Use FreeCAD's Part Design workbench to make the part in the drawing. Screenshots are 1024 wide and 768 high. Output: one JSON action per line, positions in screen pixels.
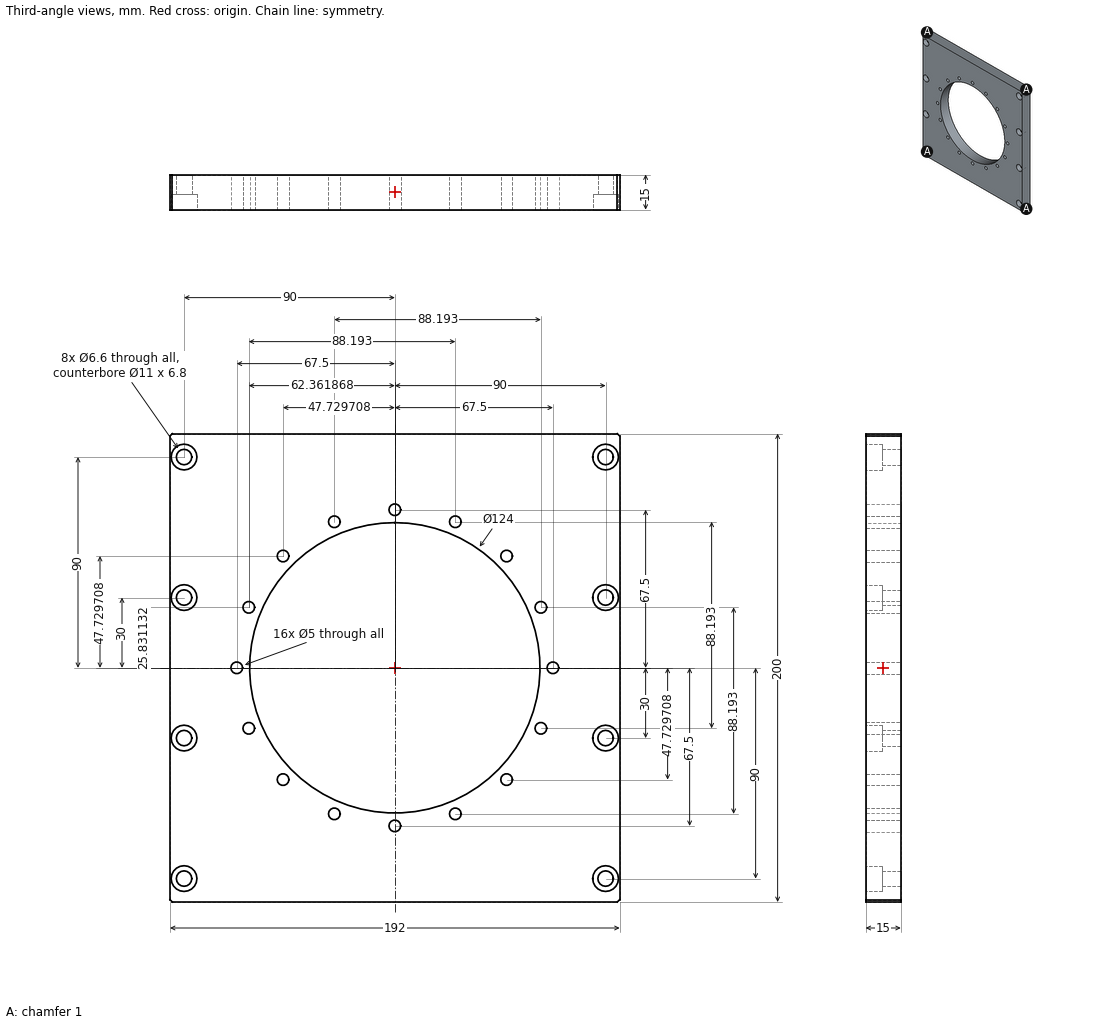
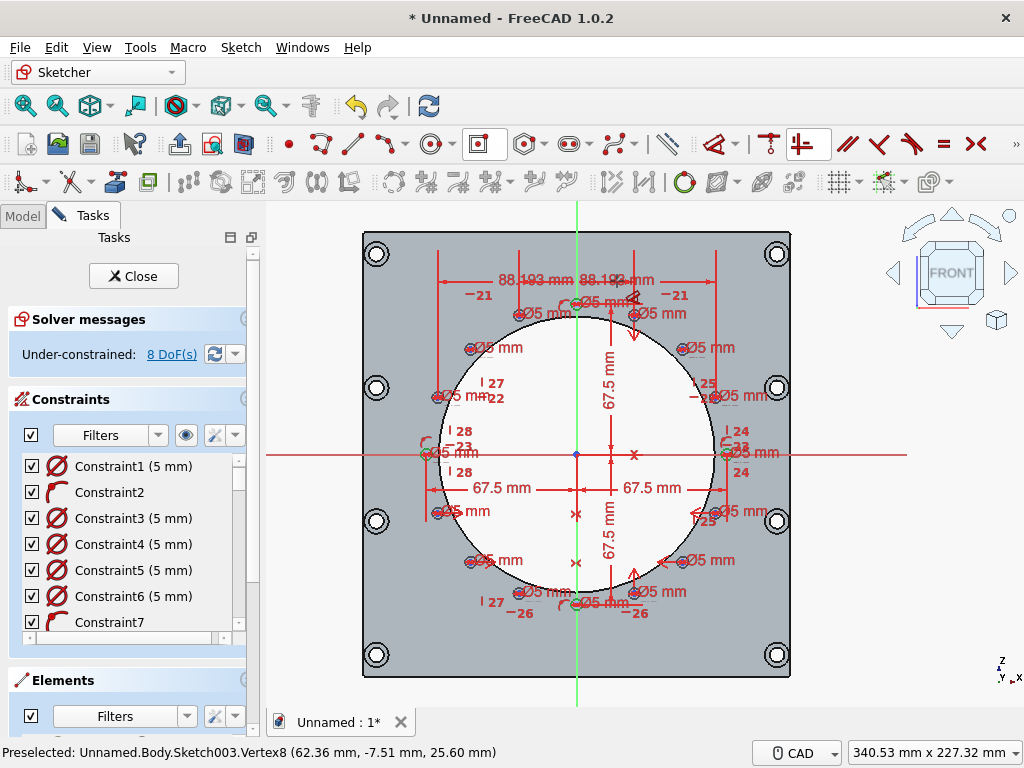
{"action": "left_click", "coordinate": [634, 315]}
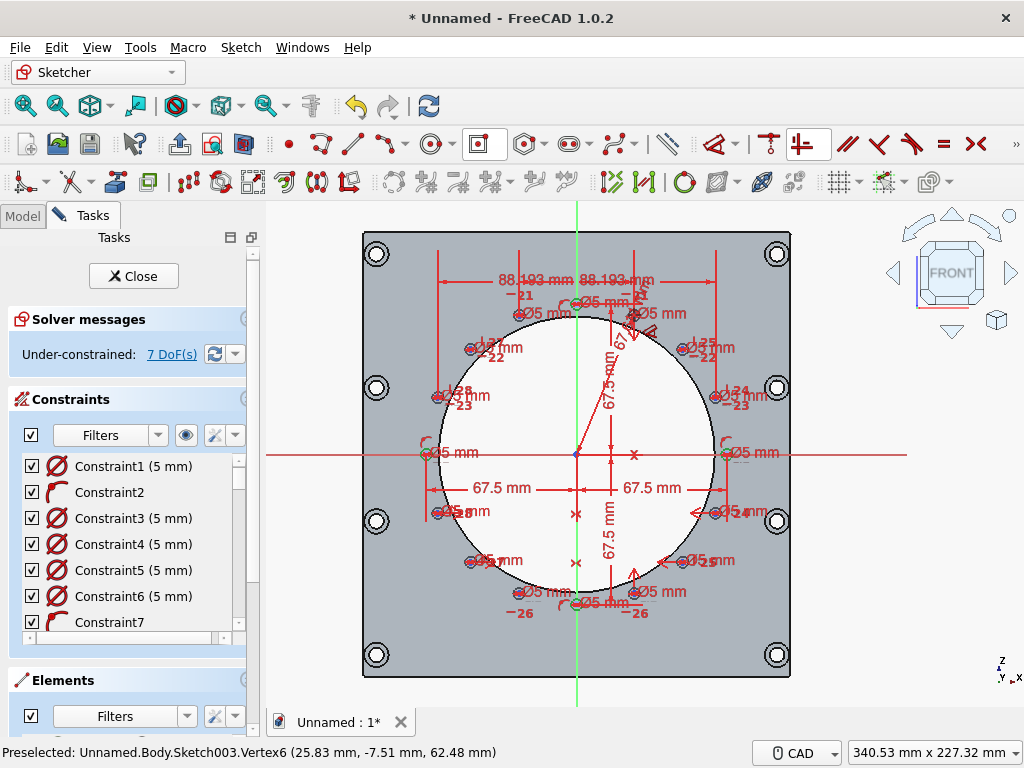
{"action": "left_click", "coordinate": [716, 513]}
{"action": "left_click", "coordinate": [750, 414]}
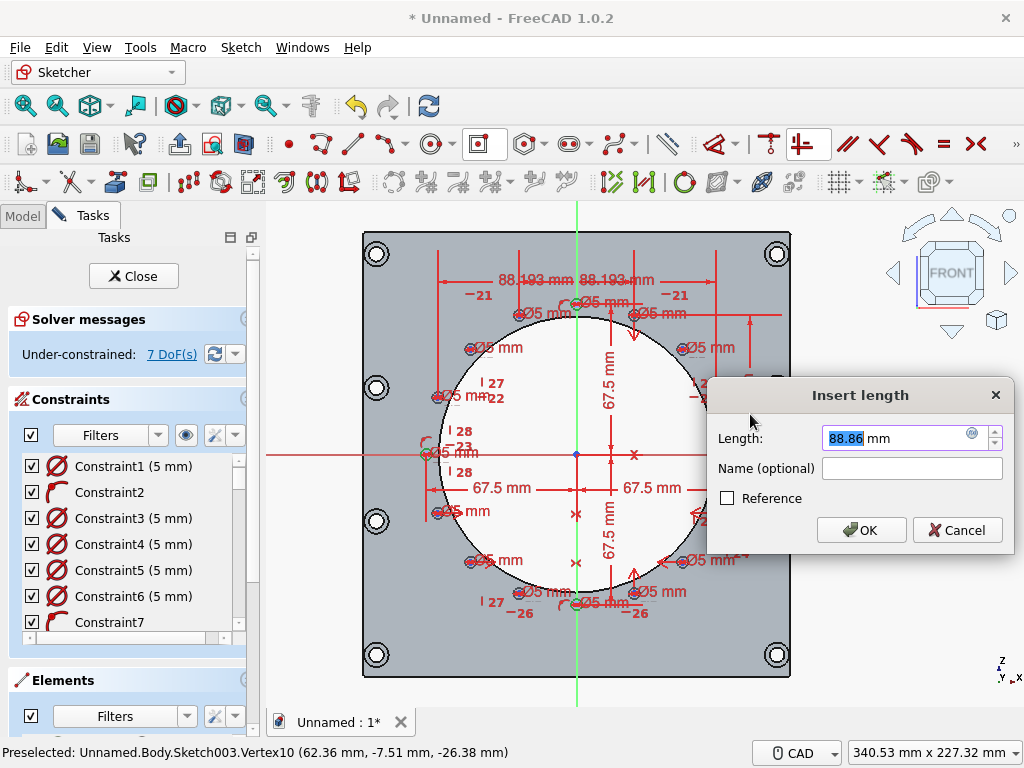
{"action": "type", "text": "88.193"}
{"action": "key", "text": "Return"}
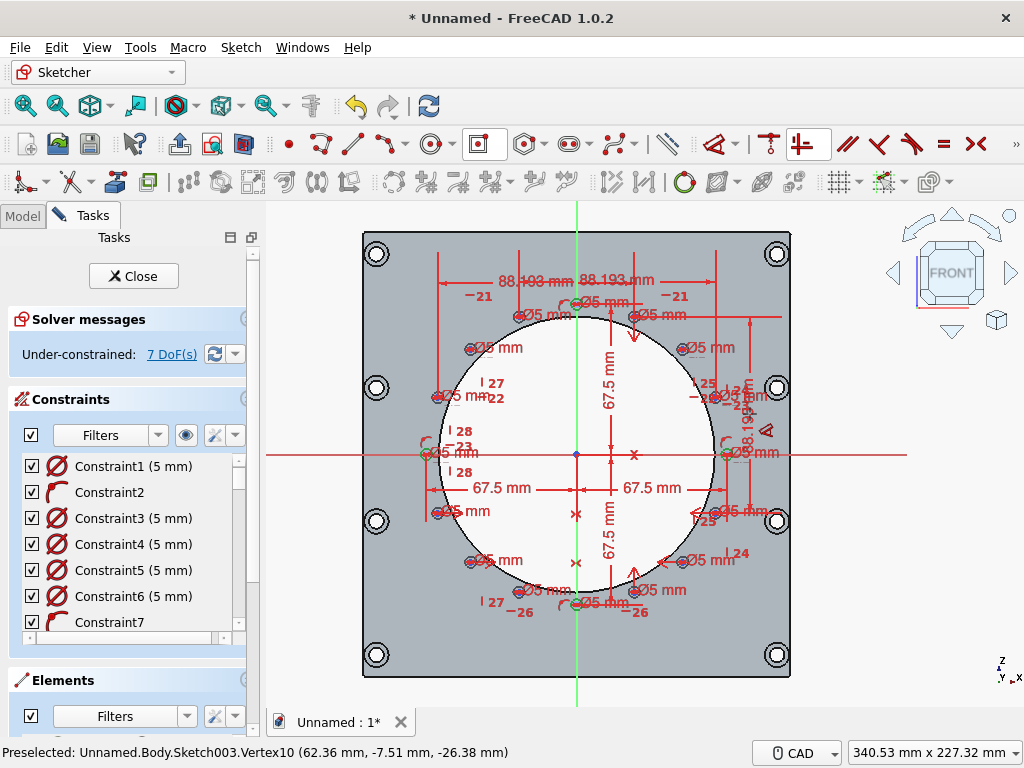
{"action": "left_click", "coordinate": [716, 398]}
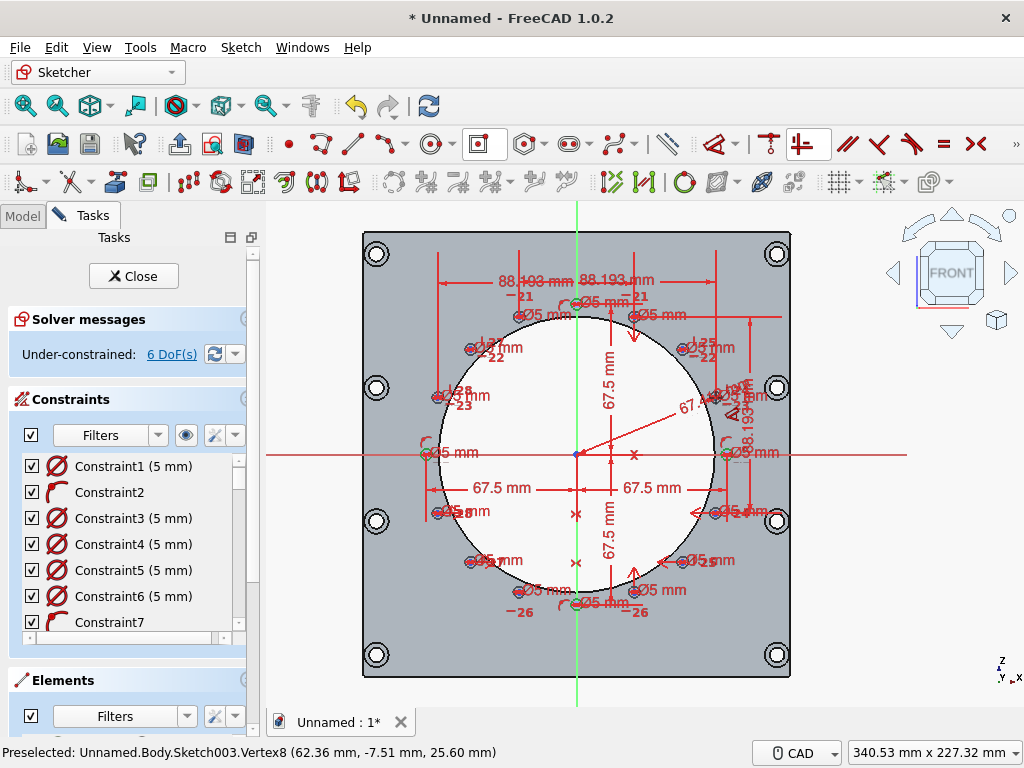
{"action": "left_click", "coordinate": [634, 592]}
{"action": "left_click", "coordinate": [750, 495]}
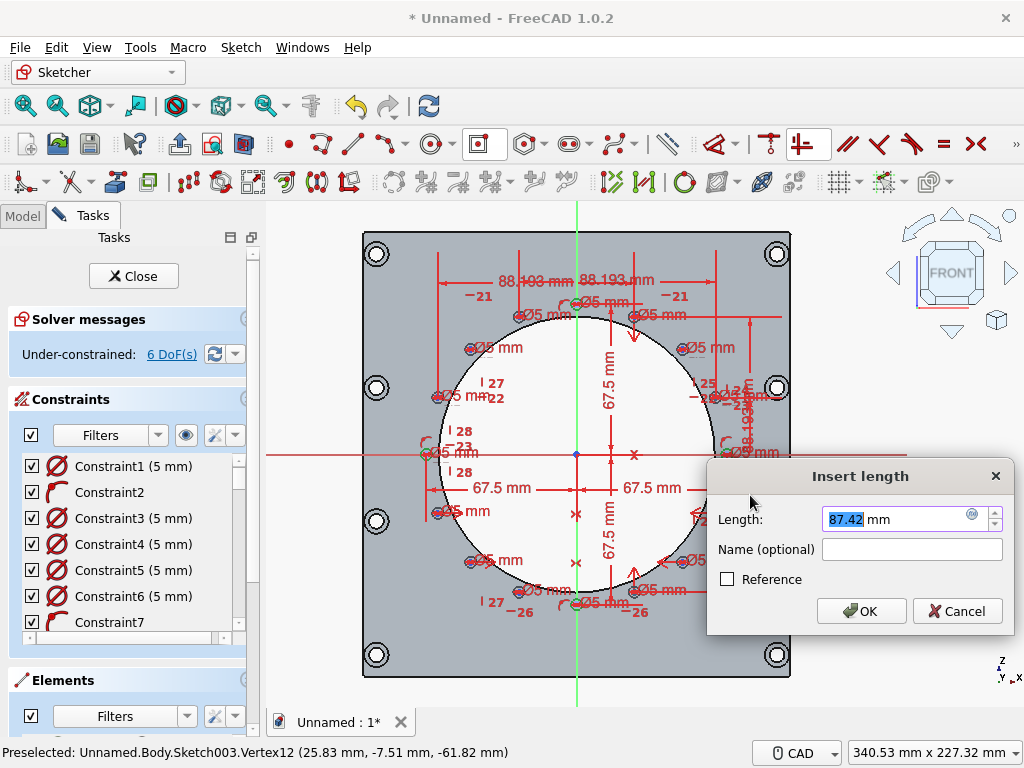
{"action": "type", "text": "88.193"}
{"action": "key", "text": "Return"}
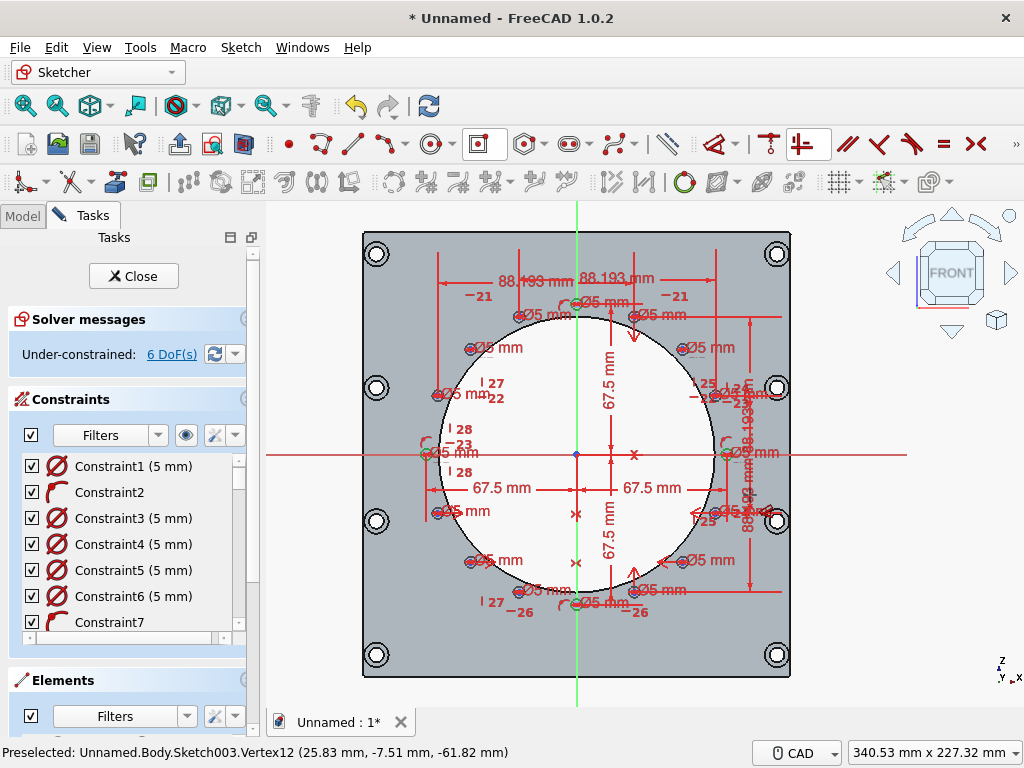
{"action": "left_click", "coordinate": [716, 513]}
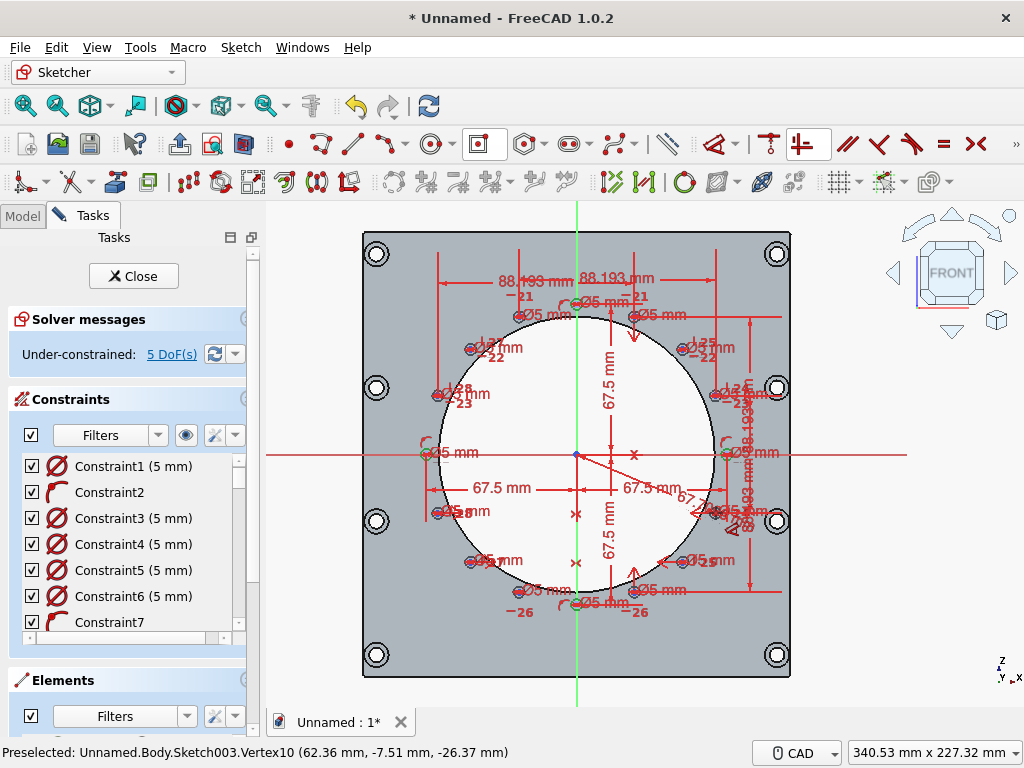
{"action": "left_click", "coordinate": [519, 592]}
{"action": "left_click", "coordinate": [617, 626]}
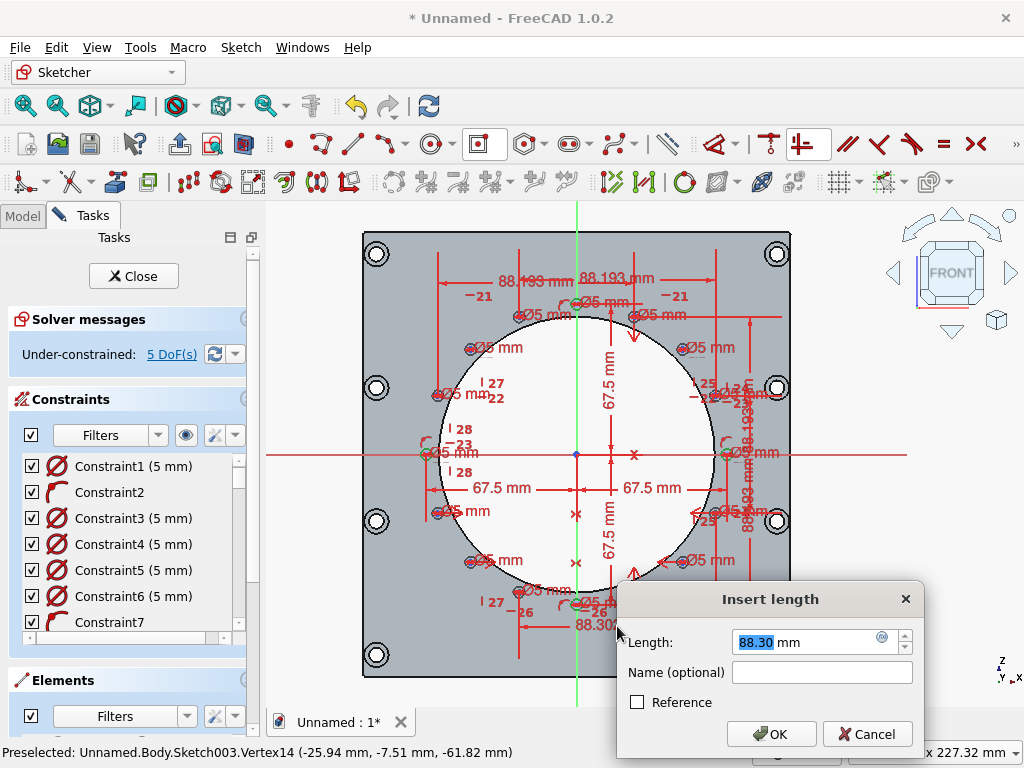
{"action": "type", "text": "88.193"}
{"action": "key", "text": "Return"}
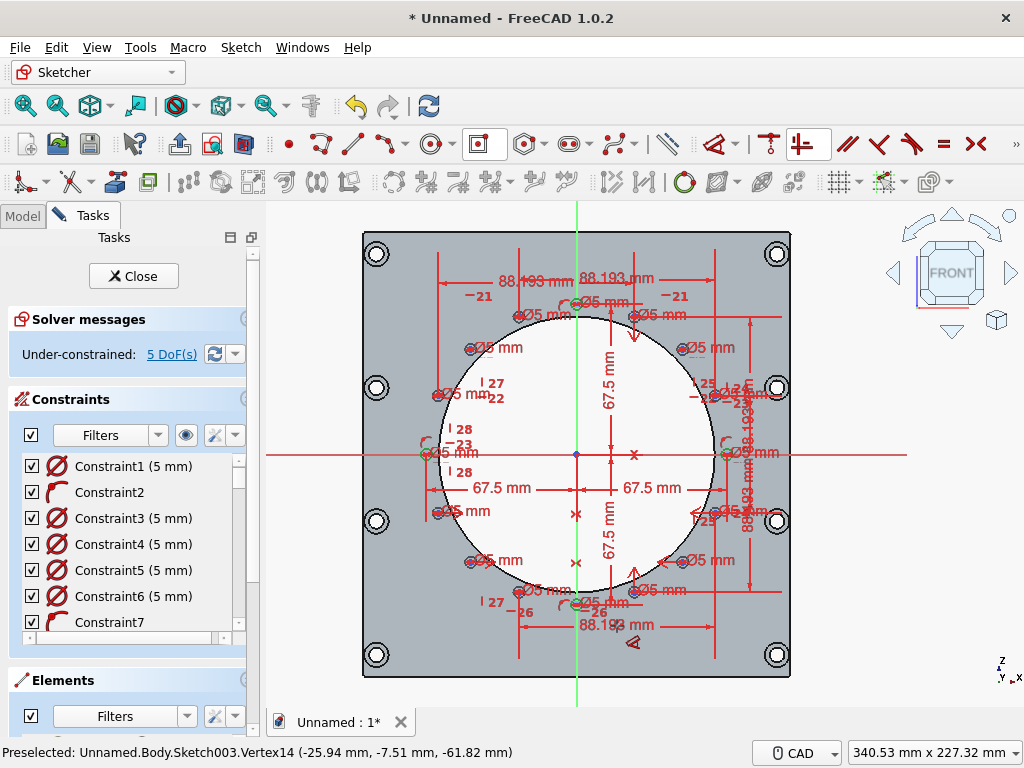
{"action": "left_click", "coordinate": [438, 396]}
{"action": "left_click", "coordinate": [507, 362]}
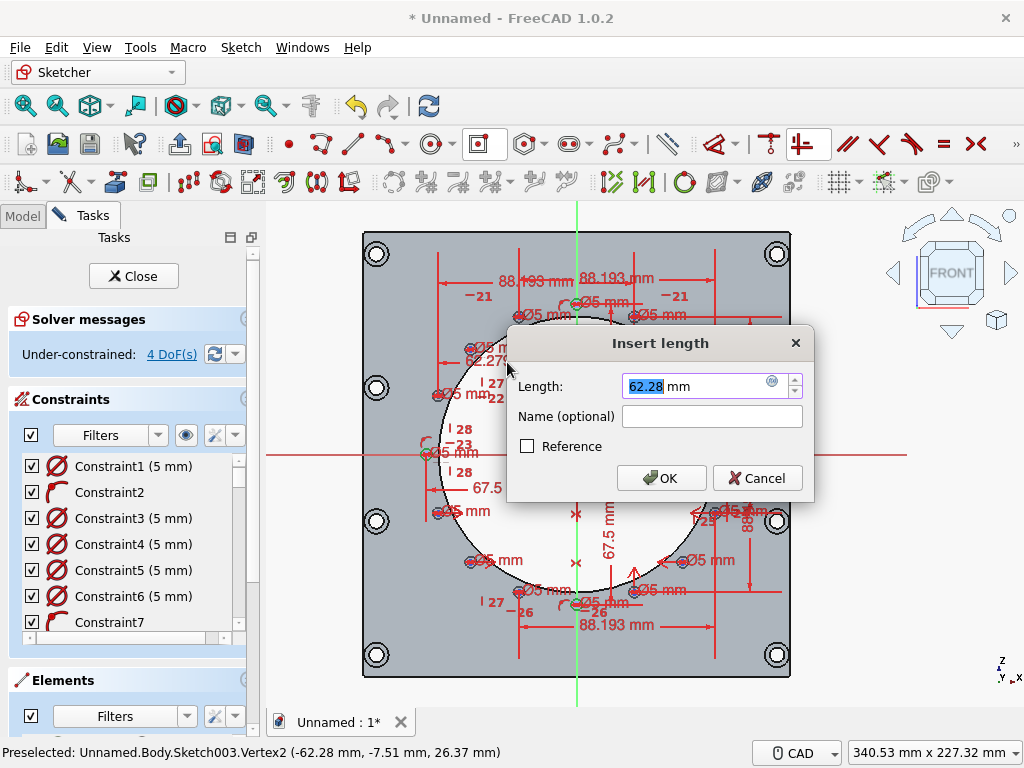
{"action": "type", "text": "62.361868"}
{"action": "key", "text": "Return"}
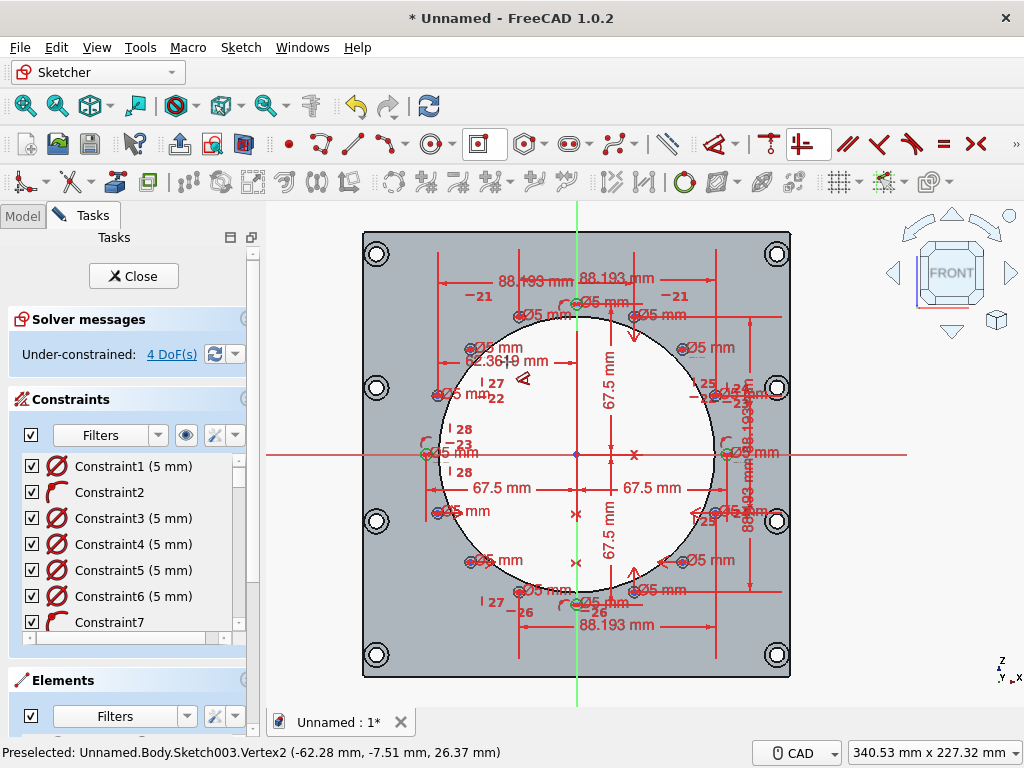
{"action": "left_click", "coordinate": [438, 396]}
{"action": "left_click", "coordinate": [404, 425]}